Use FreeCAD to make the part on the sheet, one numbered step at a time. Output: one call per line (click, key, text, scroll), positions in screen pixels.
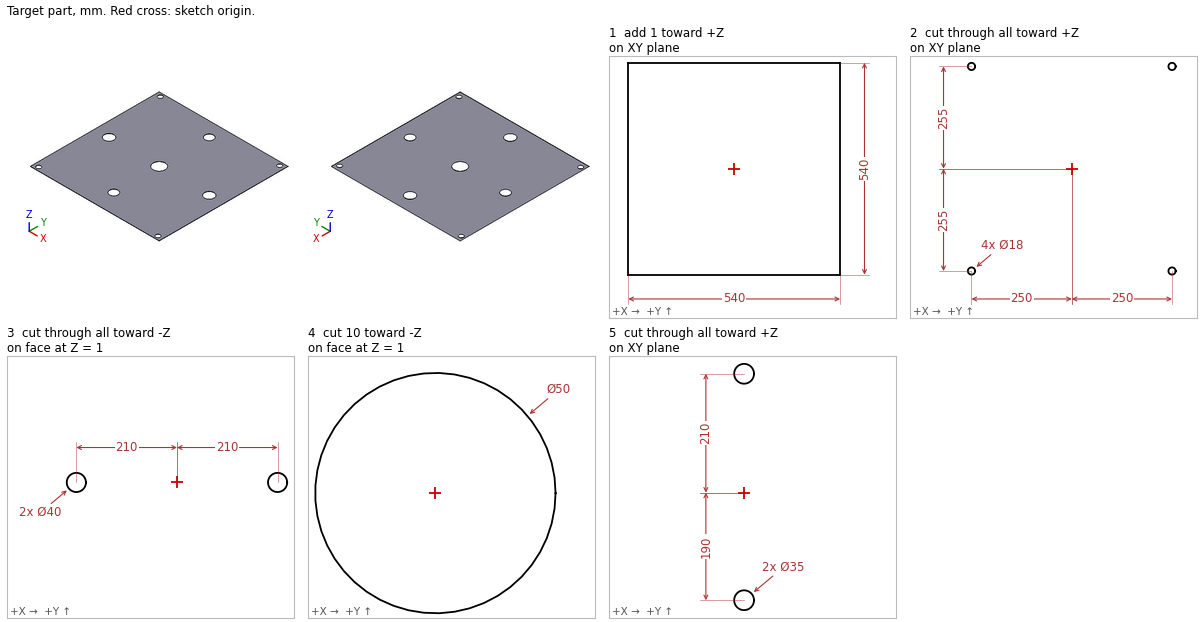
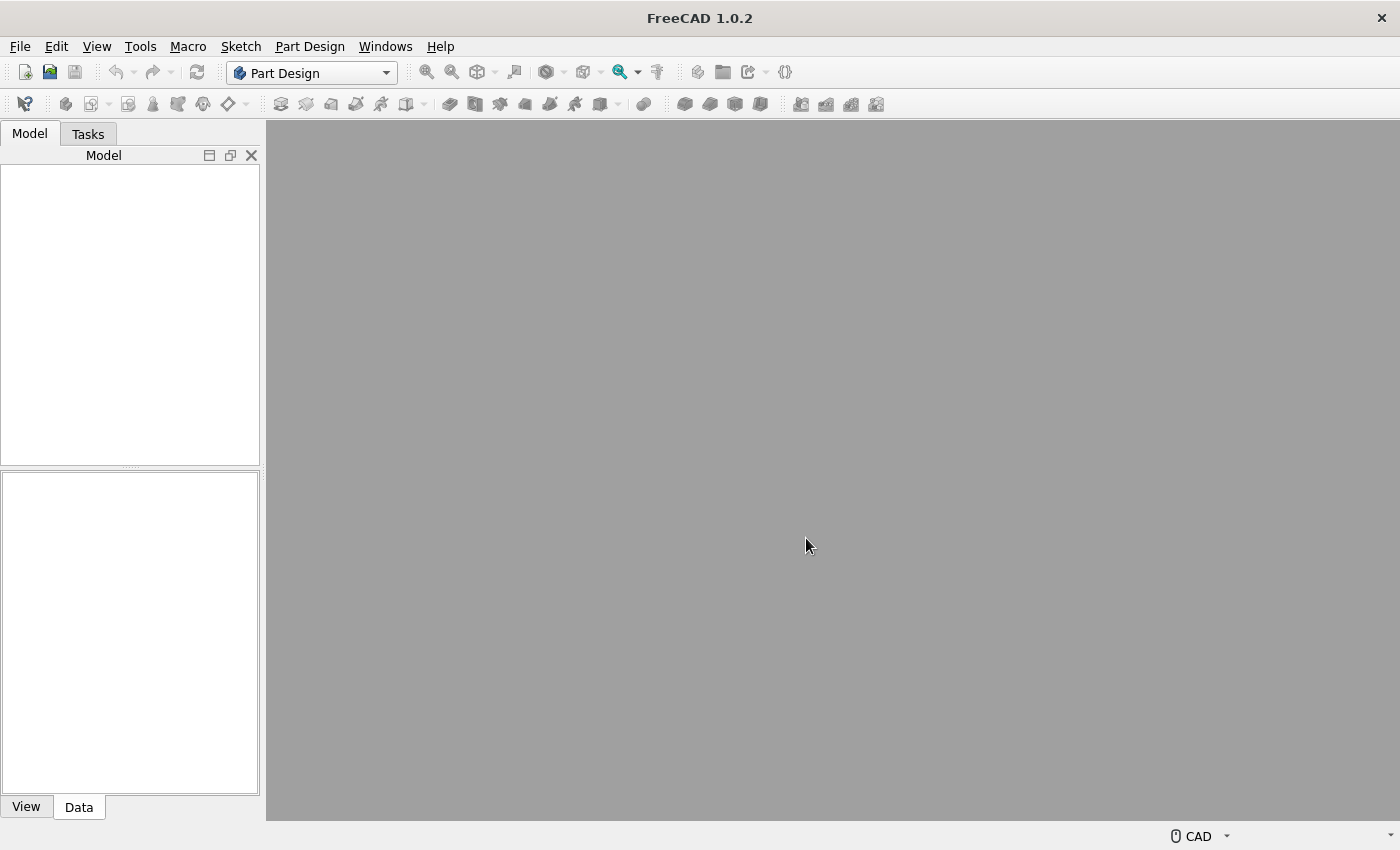
click(25, 72)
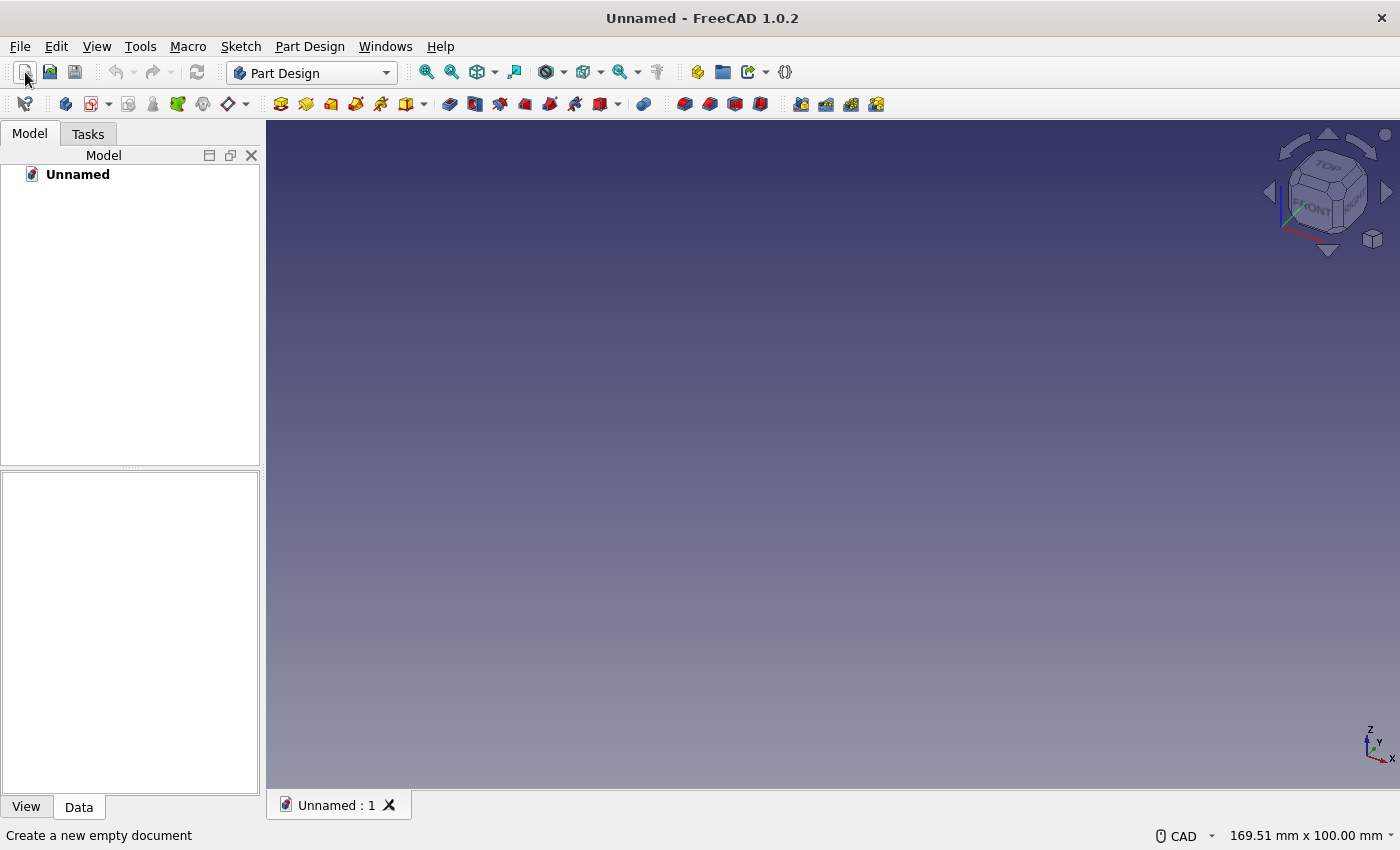
click(90, 104)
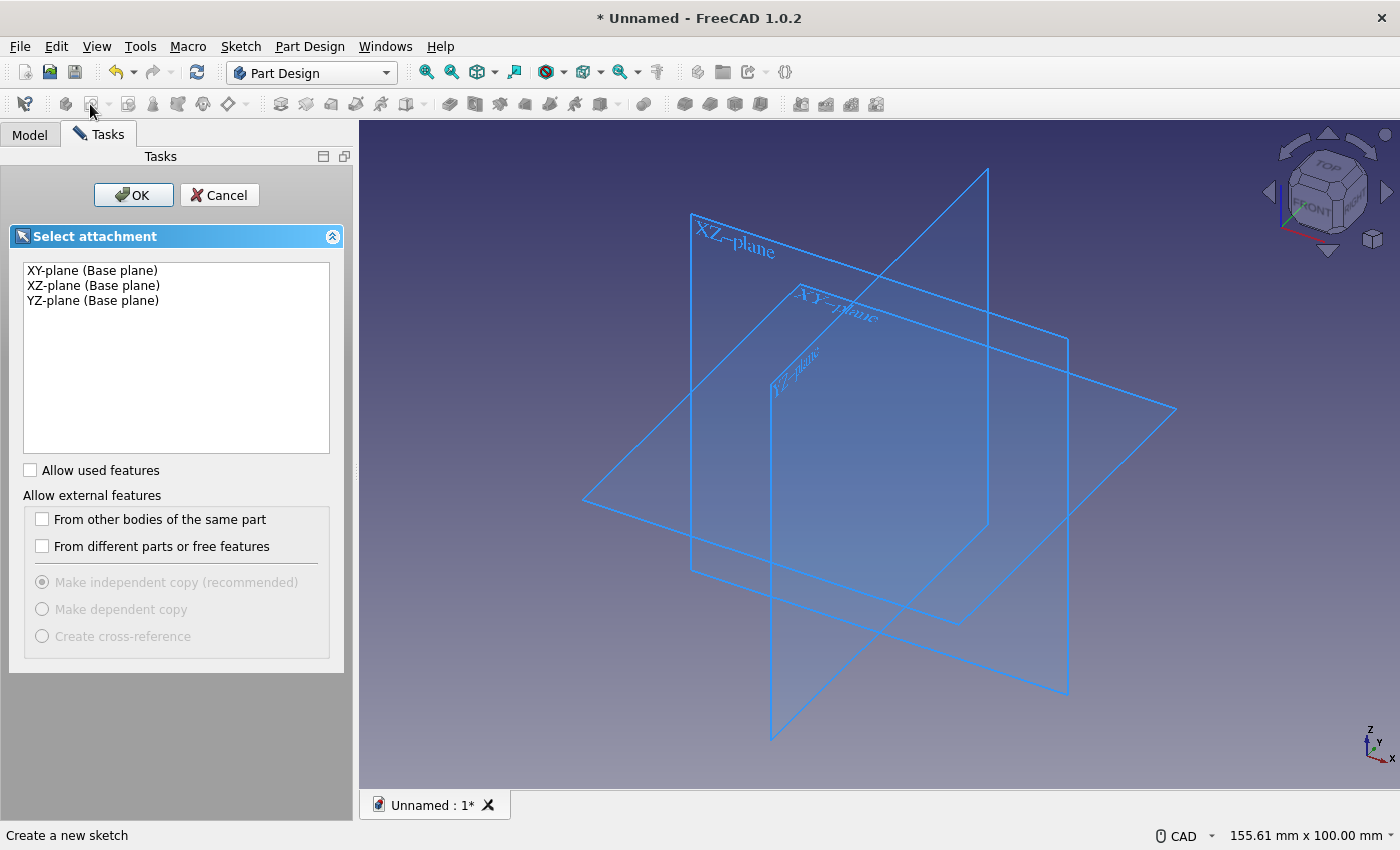
click(84, 270)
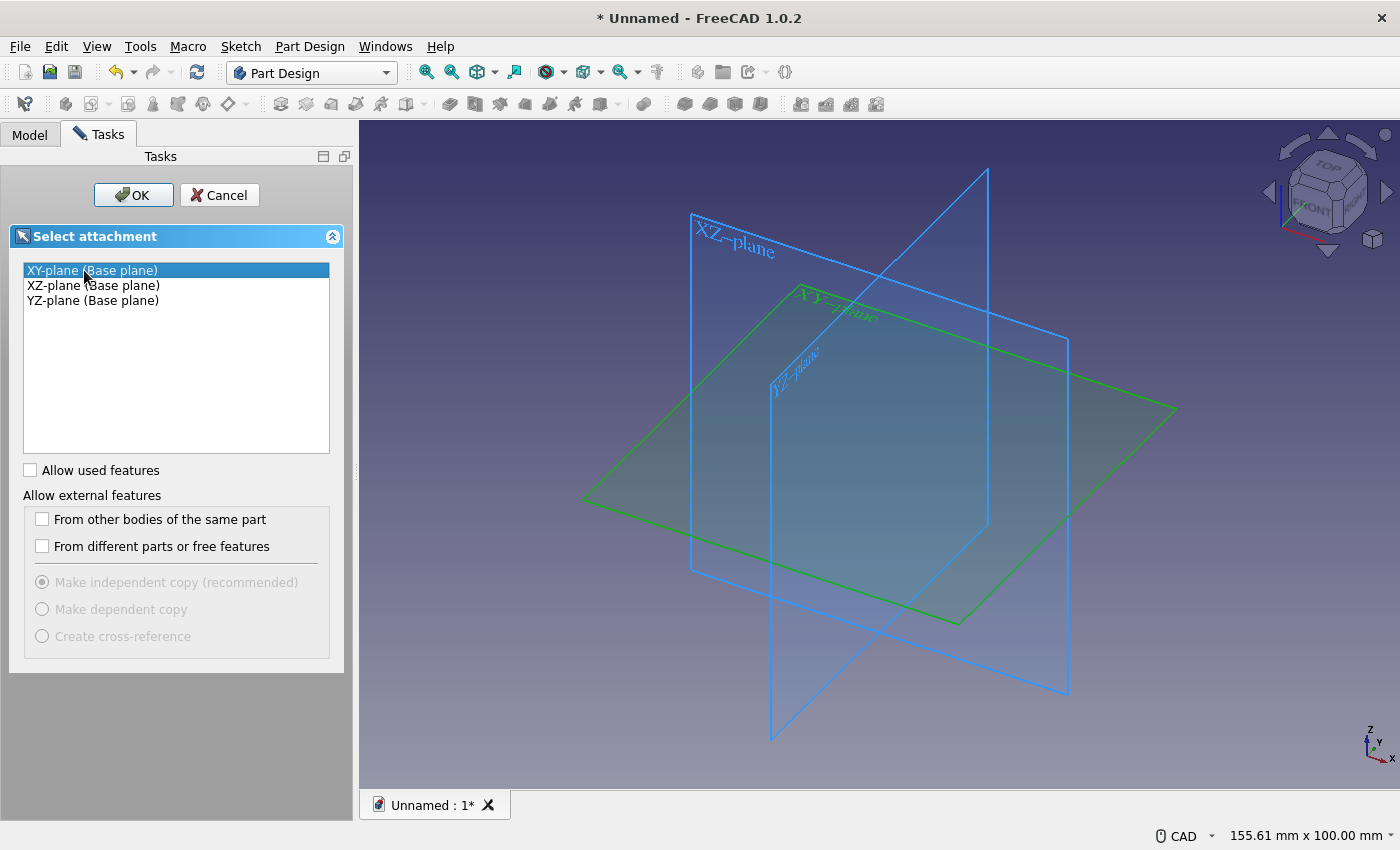
click(134, 195)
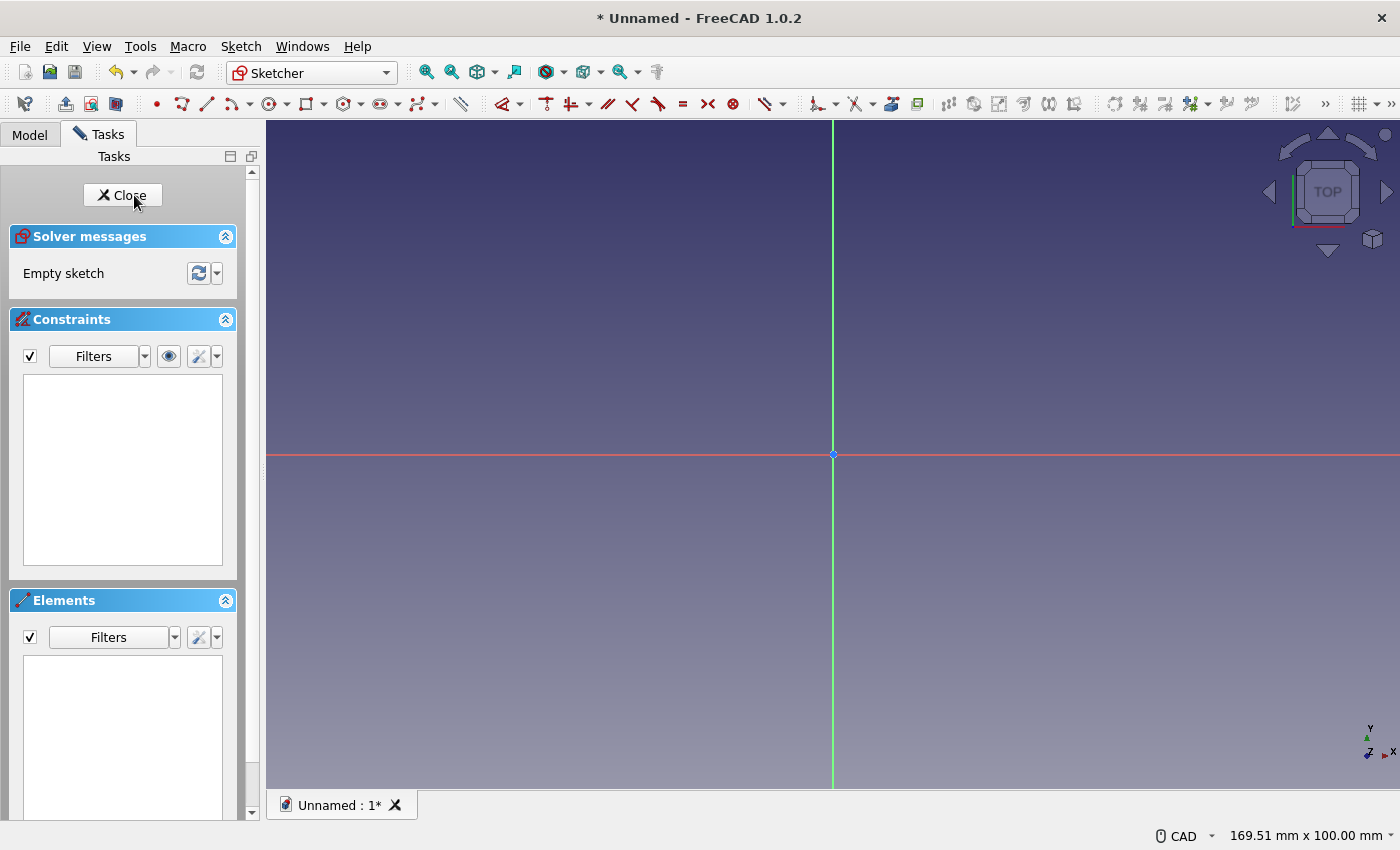
scroll(756, 454, down, 11)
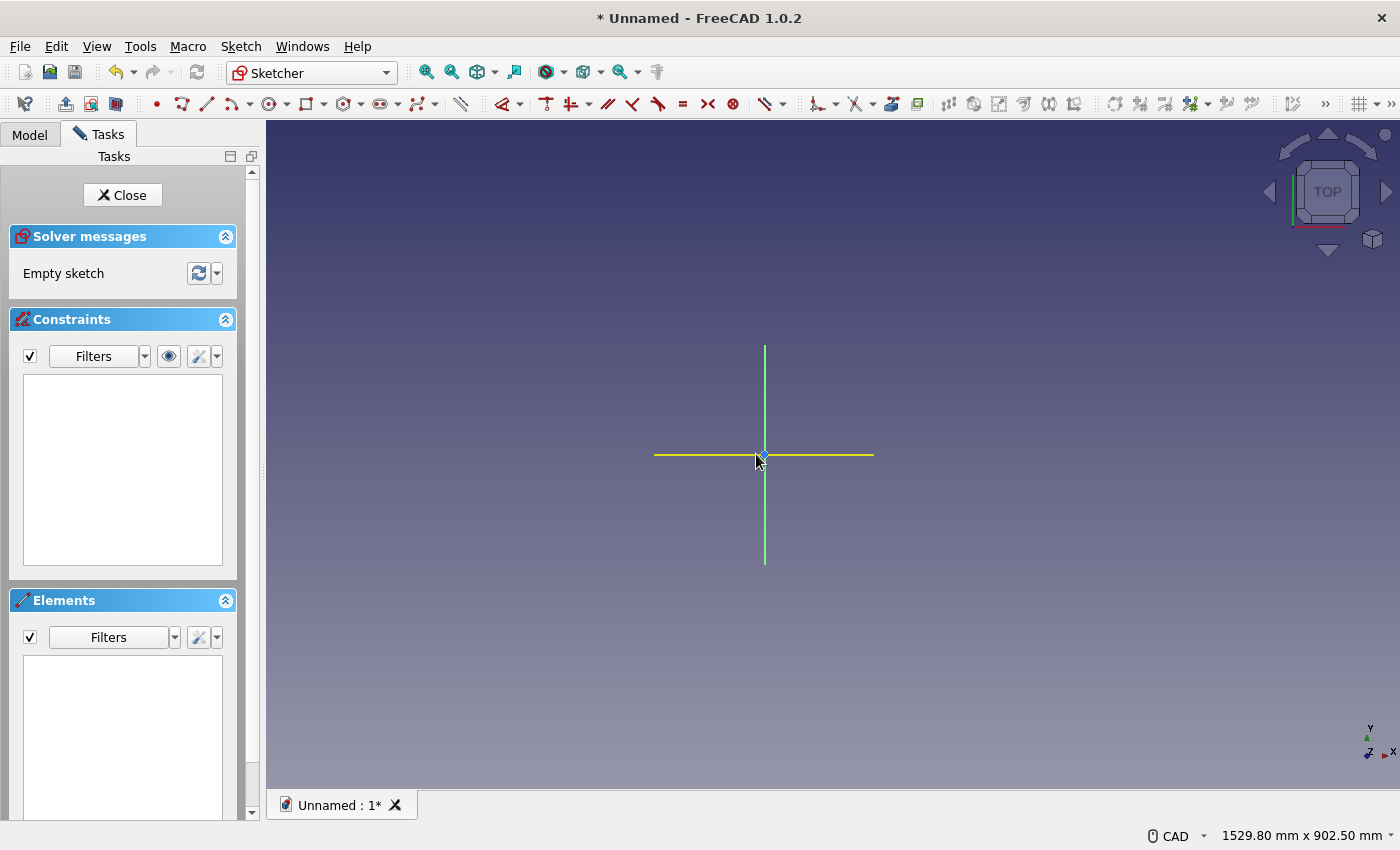
key(g)
key(v)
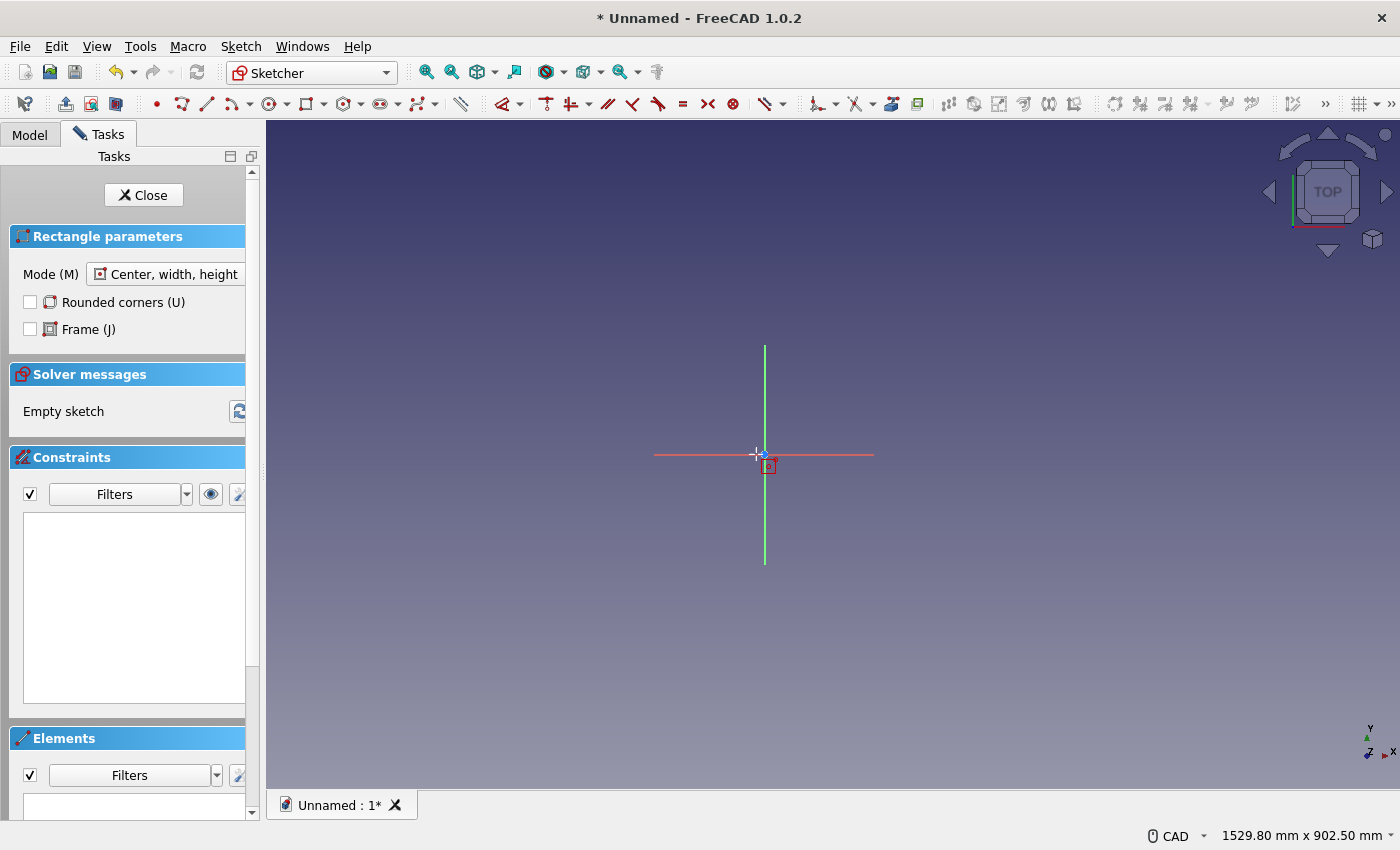
click(765, 454)
move(965, 254)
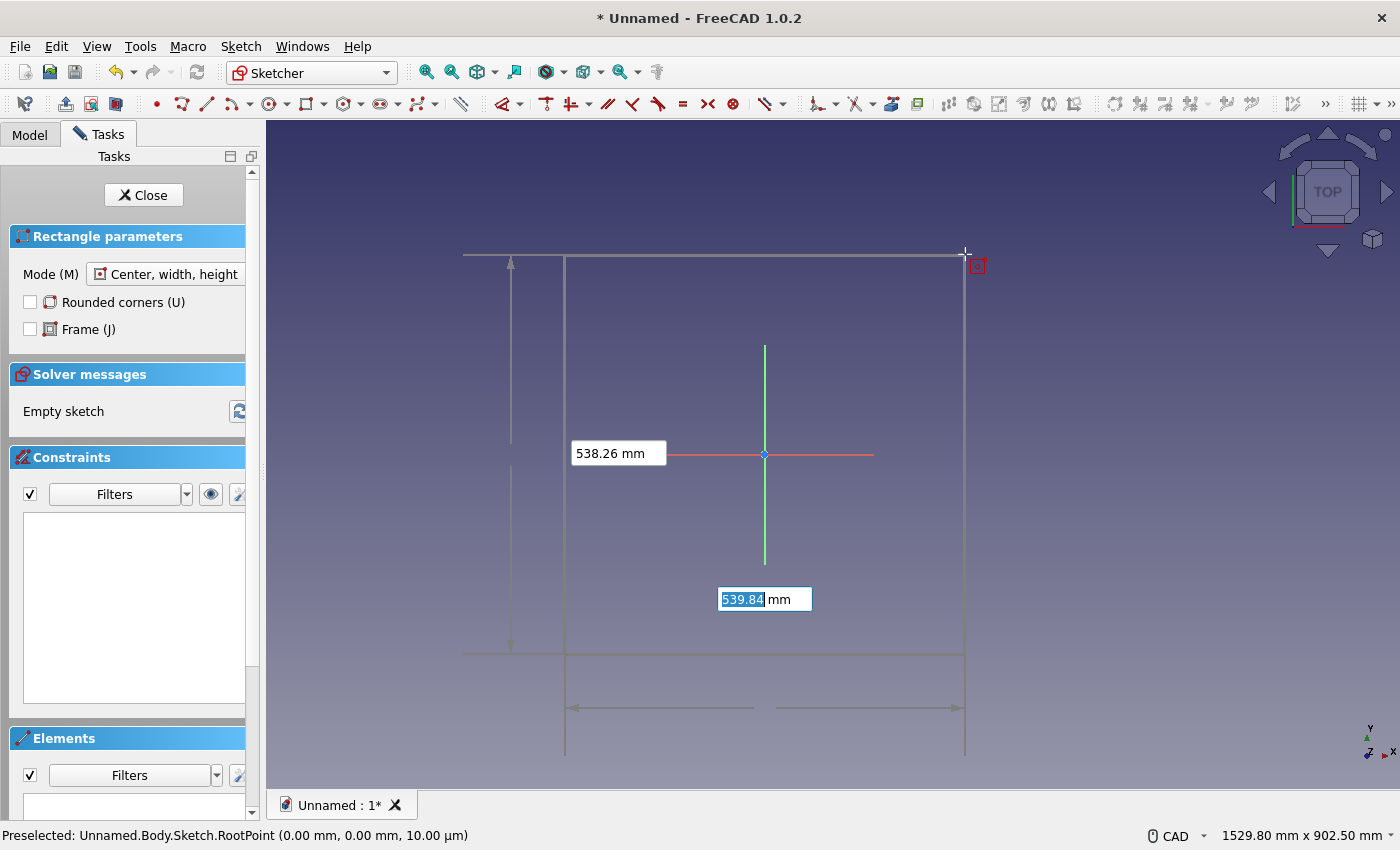
text(540)
key(Tab)
text(540)
key(Return)
key(Escape)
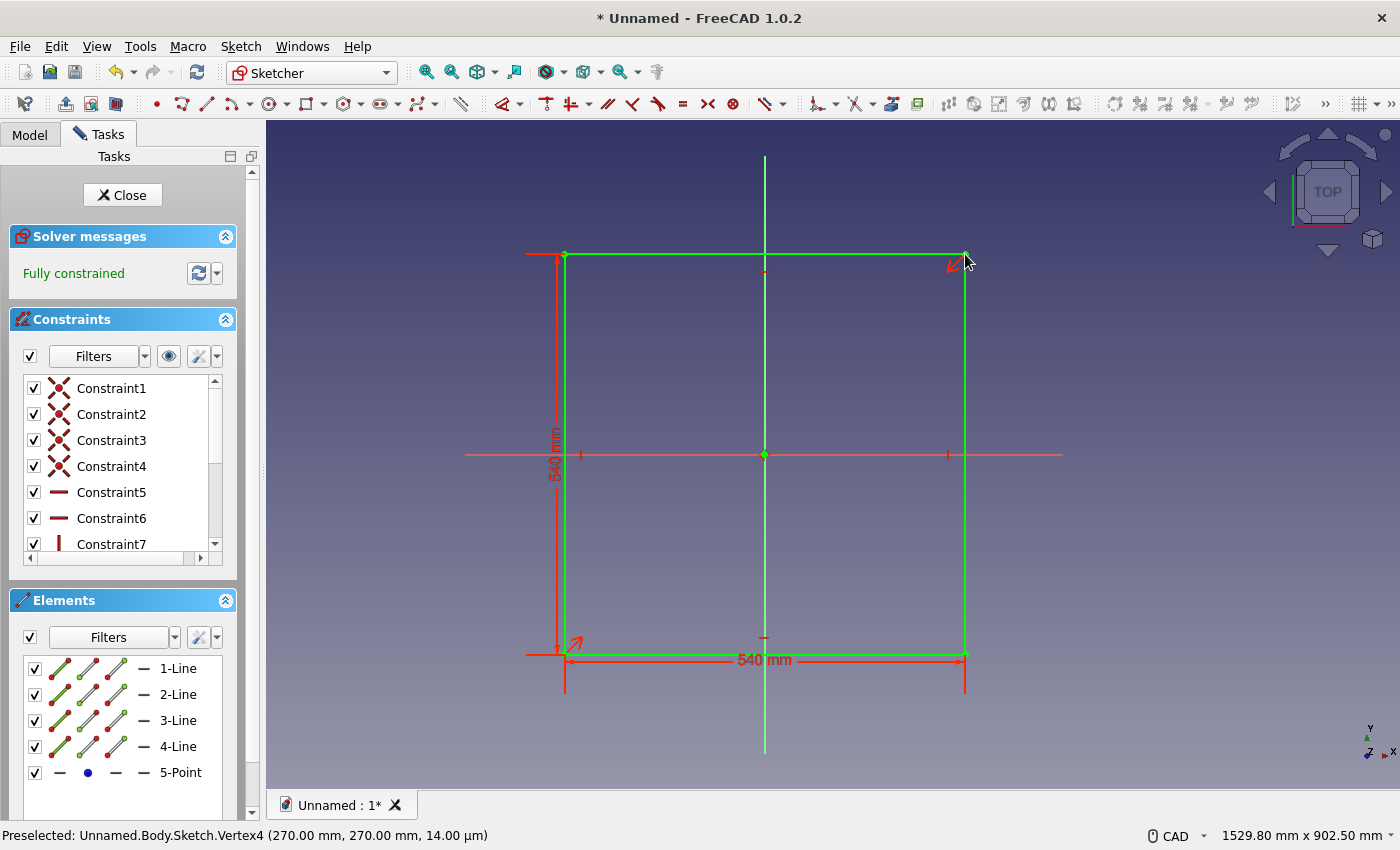
click(123, 195)